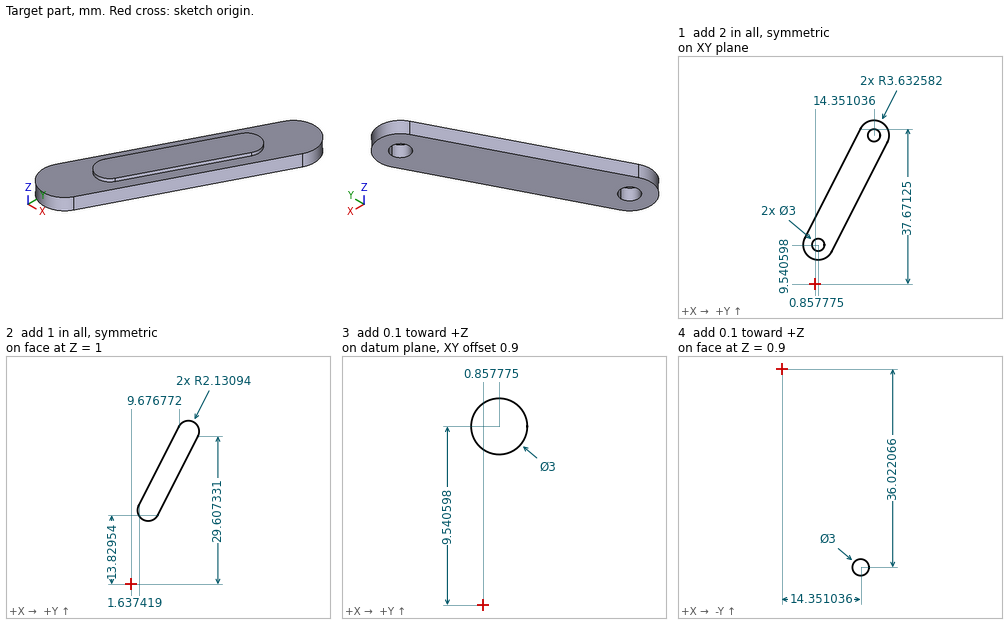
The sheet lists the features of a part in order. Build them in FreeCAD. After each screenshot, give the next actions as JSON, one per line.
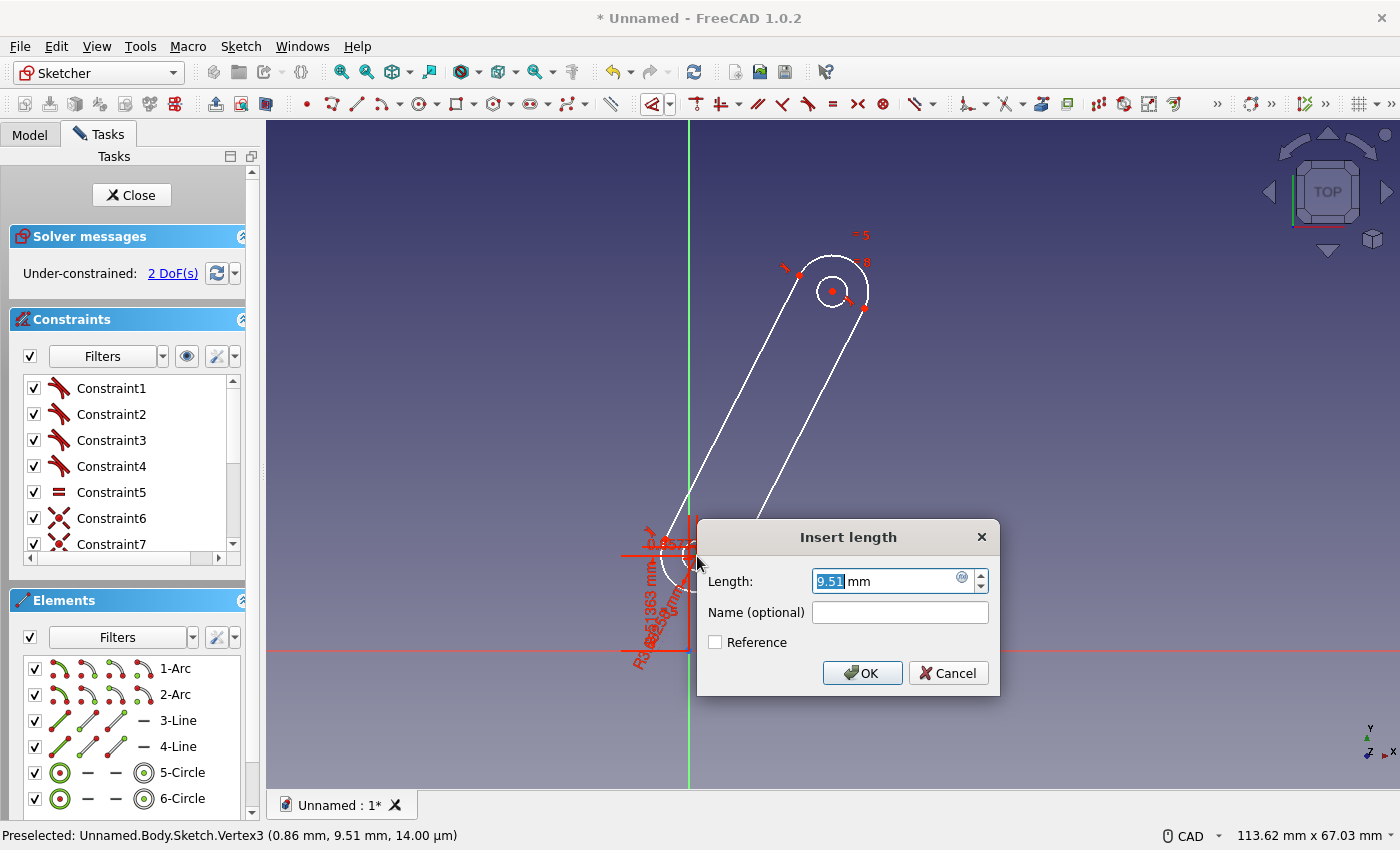
{"action": "type", "text": "9.540598"}
{"action": "key", "text": "Return"}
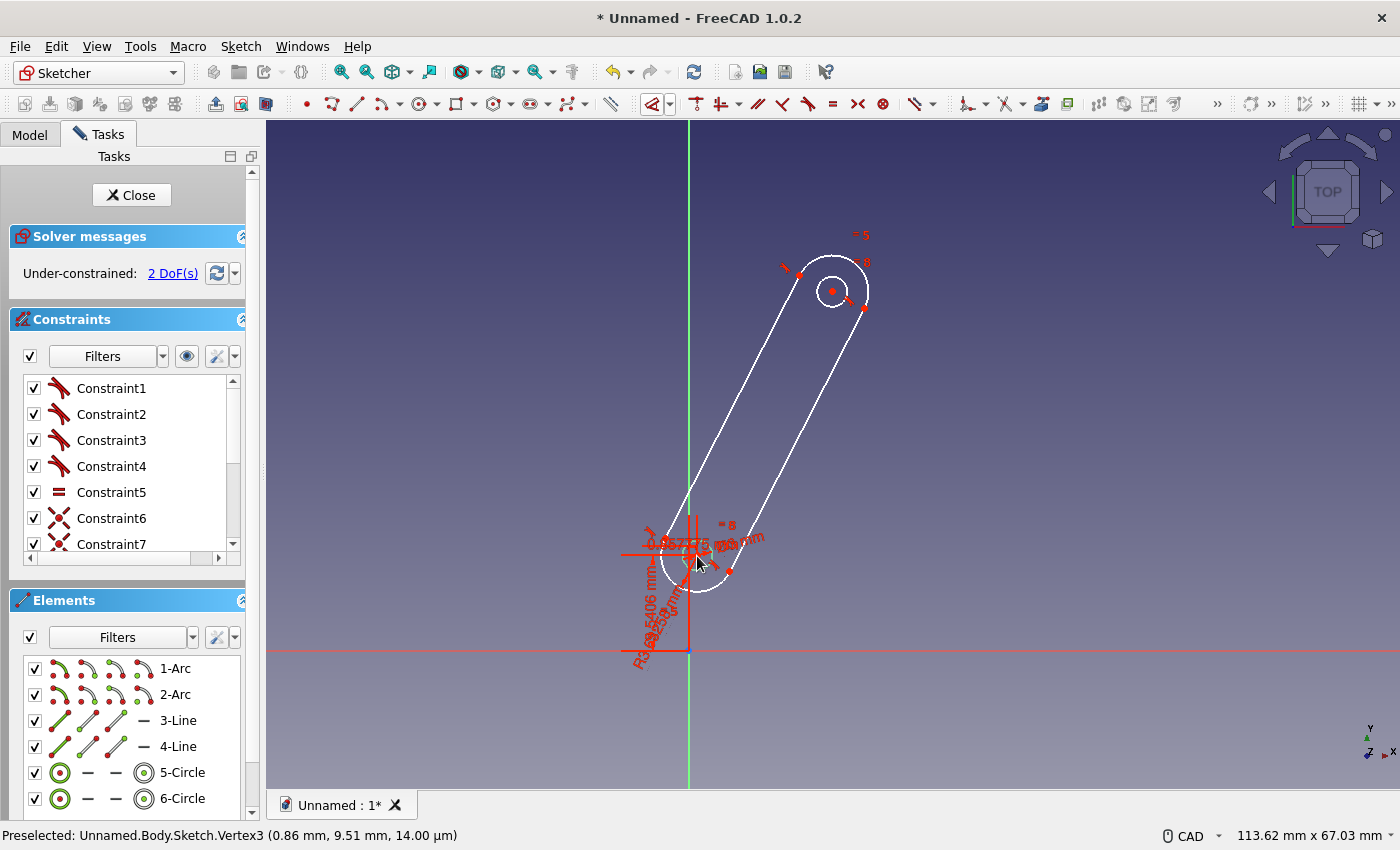
{"action": "left_click", "coordinate": [800, 275]}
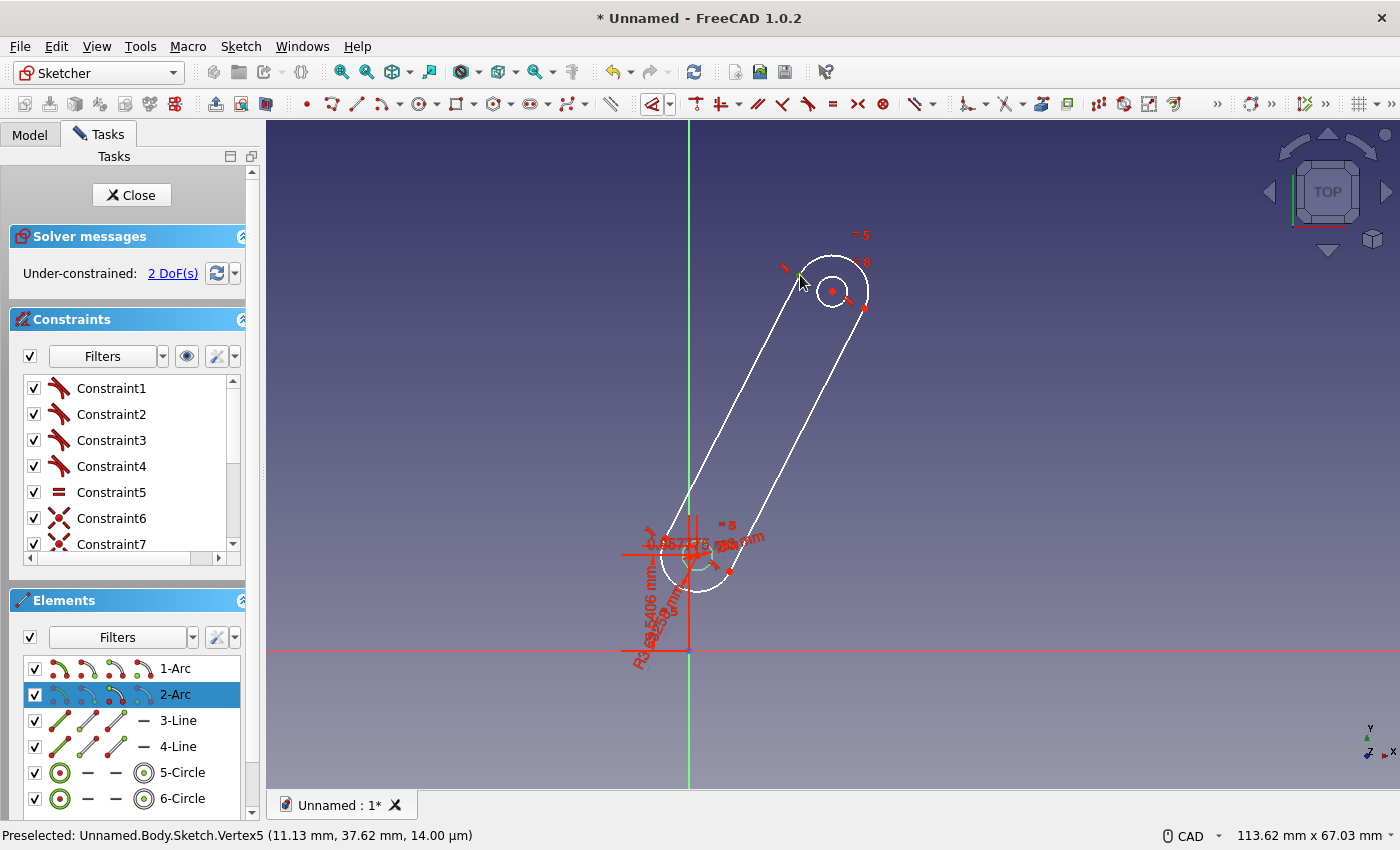
{"action": "key", "text": "i"}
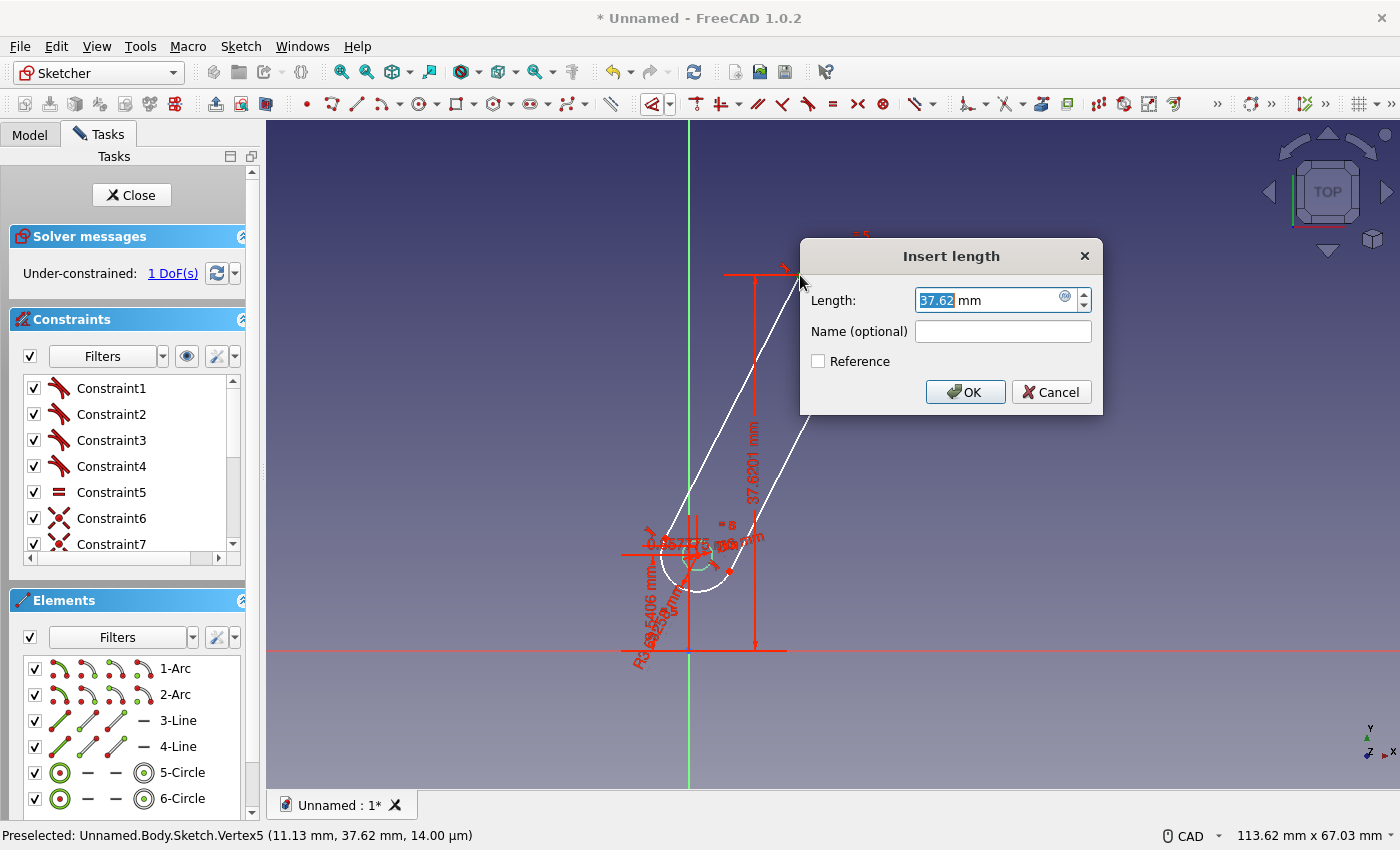
{"action": "type", "text": "37.67125"}
{"action": "key", "text": "Return"}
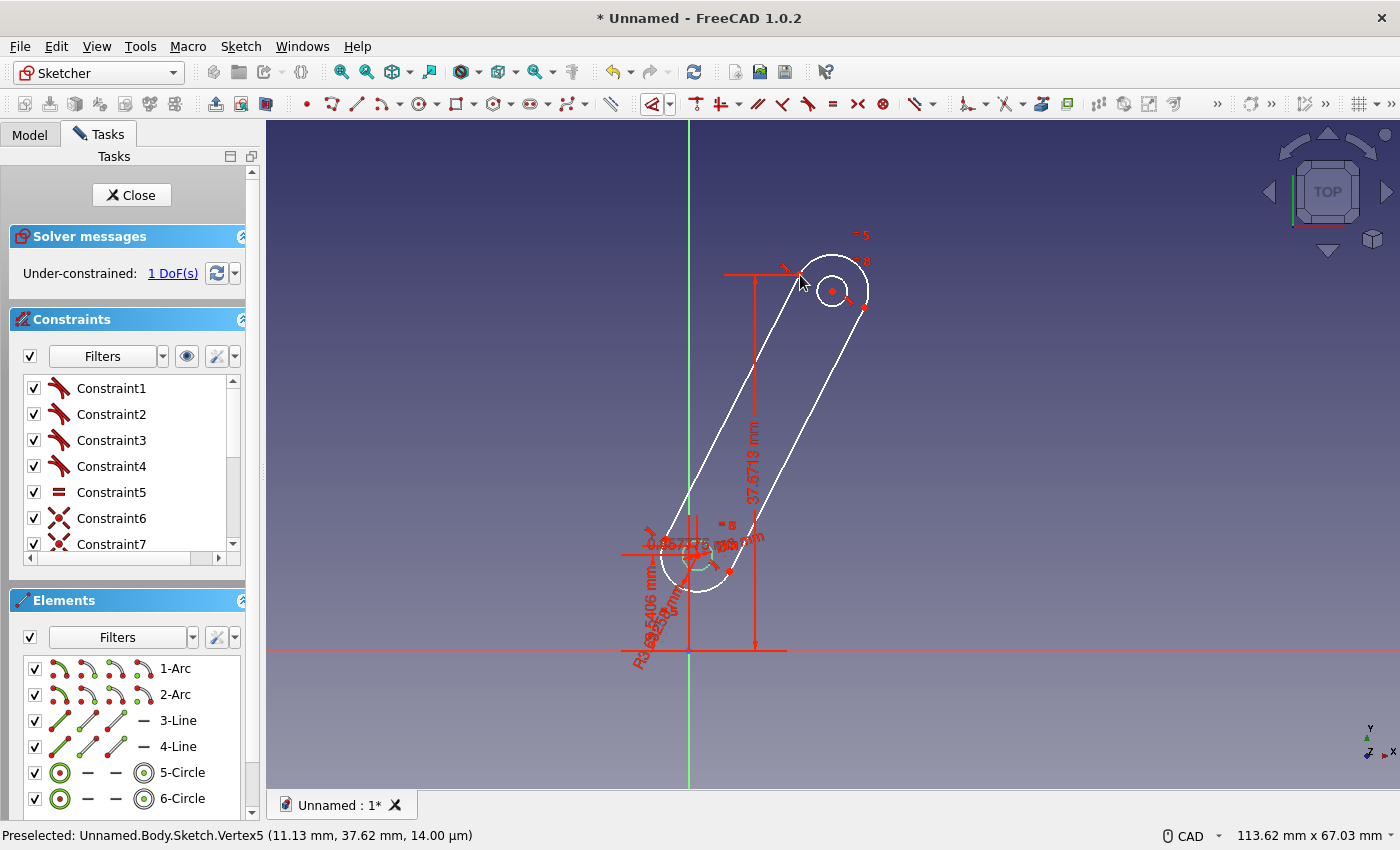
{"action": "left_click", "coordinate": [832, 291]}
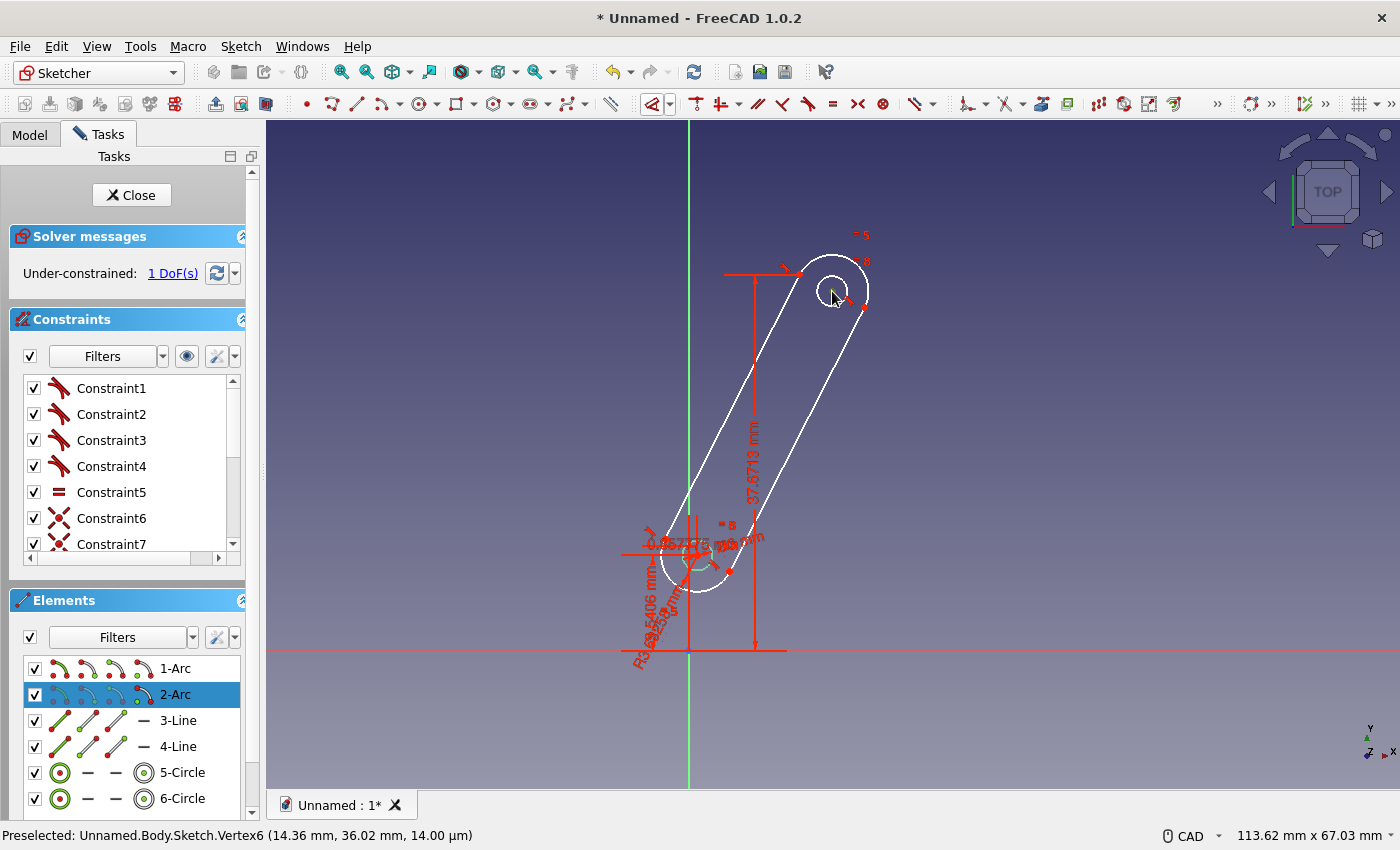
{"action": "key", "text": "l"}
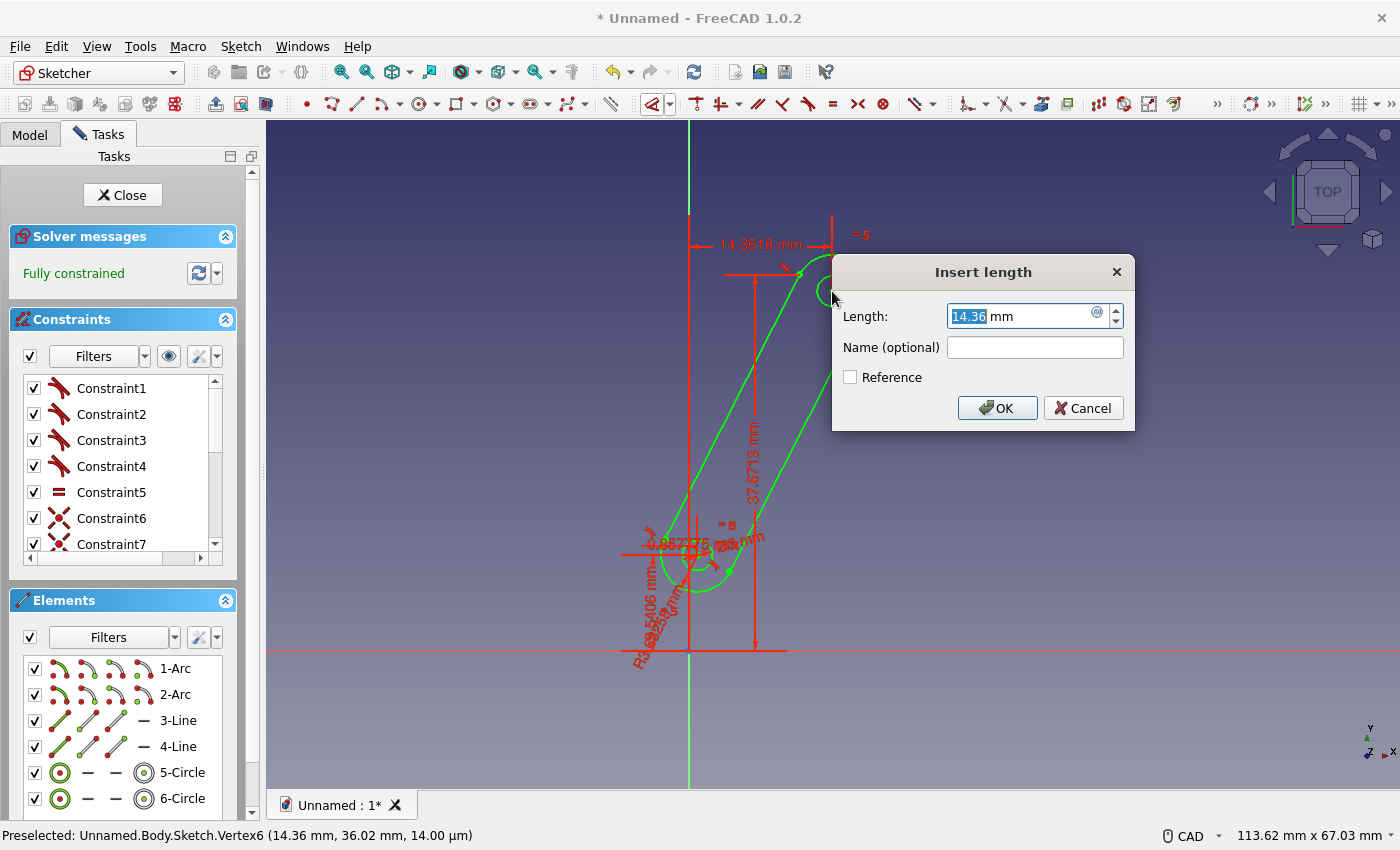
{"action": "type", "text": "14.351036"}
{"action": "key", "text": "Return"}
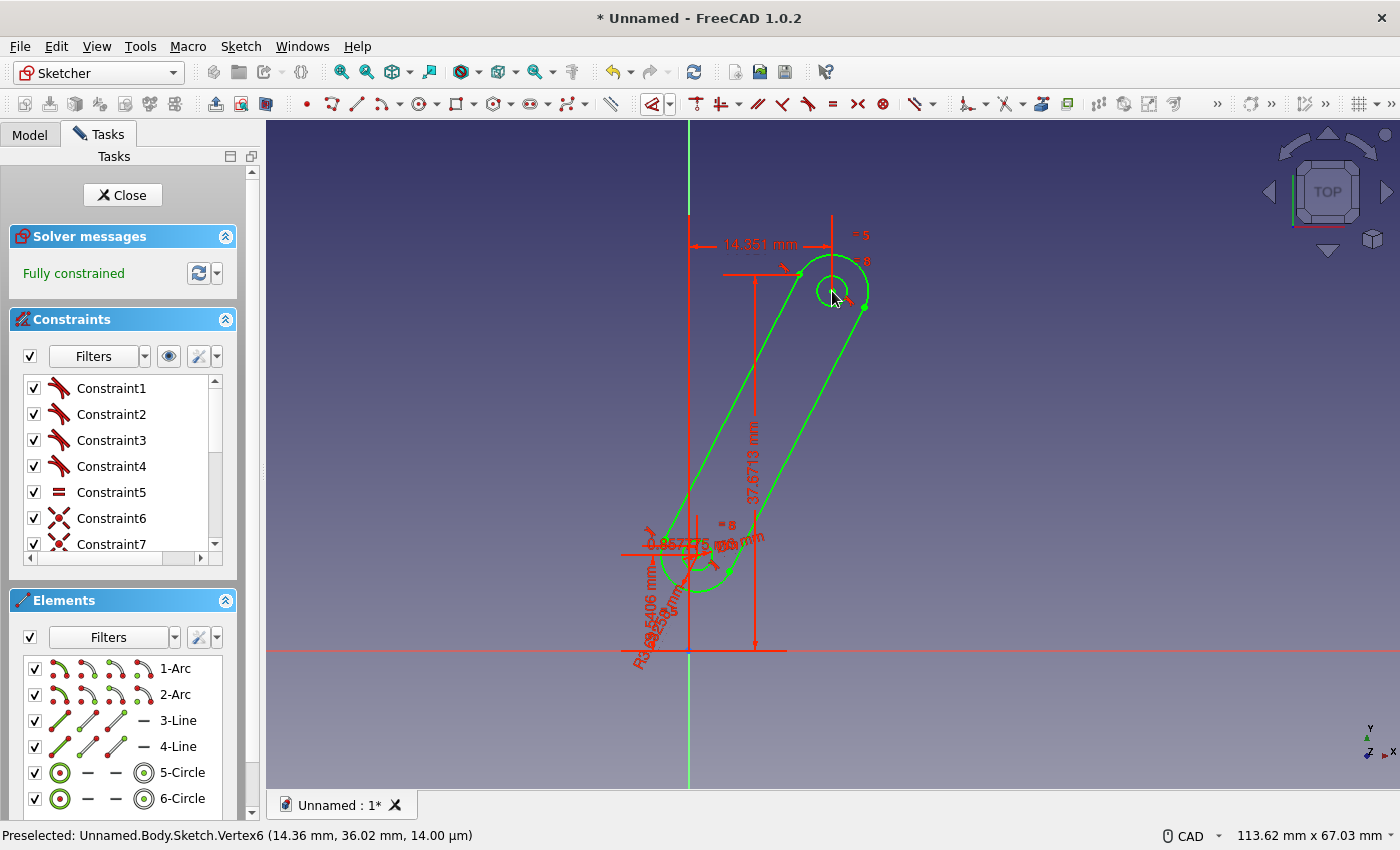
{"action": "left_click", "coordinate": [123, 195]}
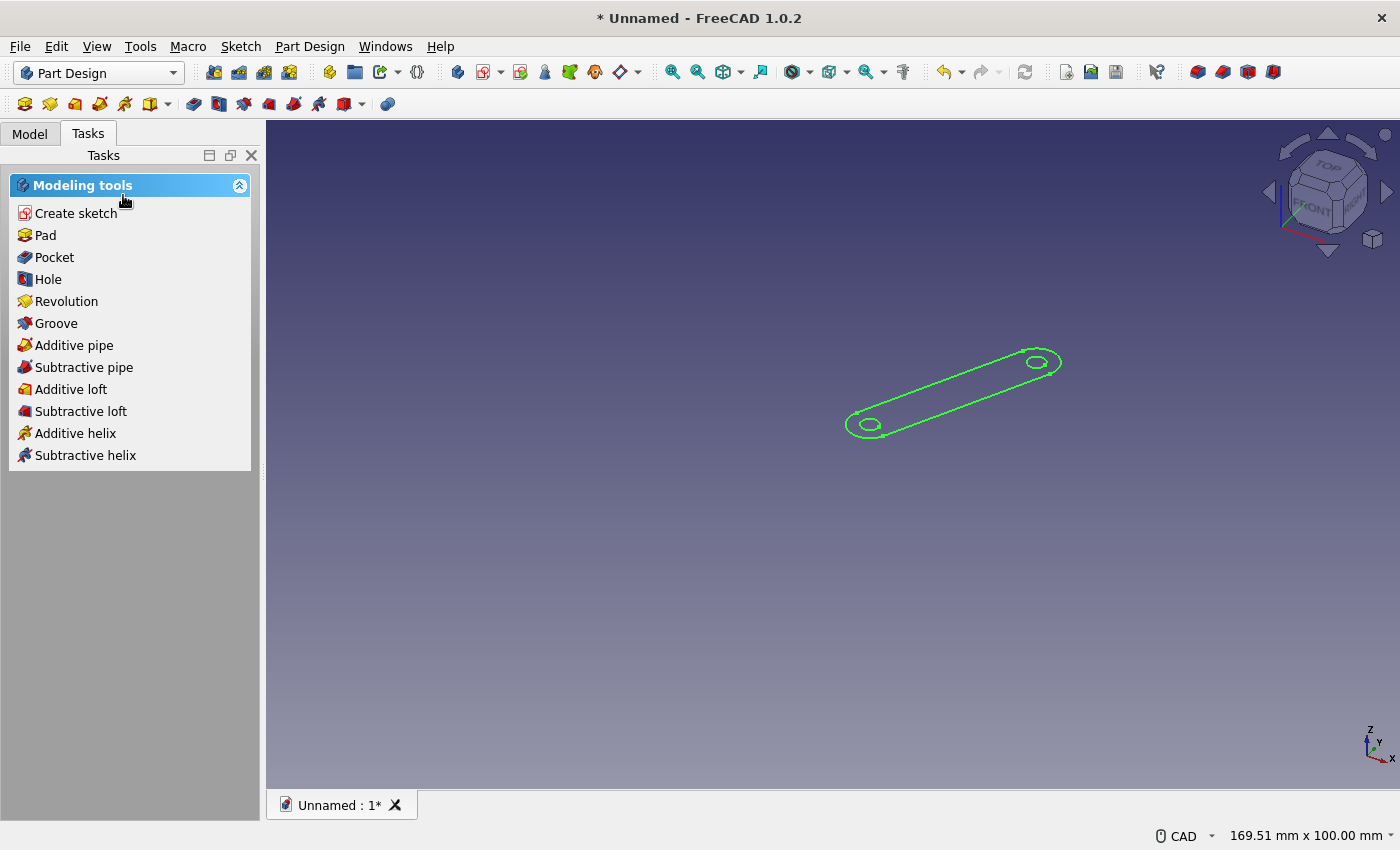
{"action": "left_click", "coordinate": [25, 104]}